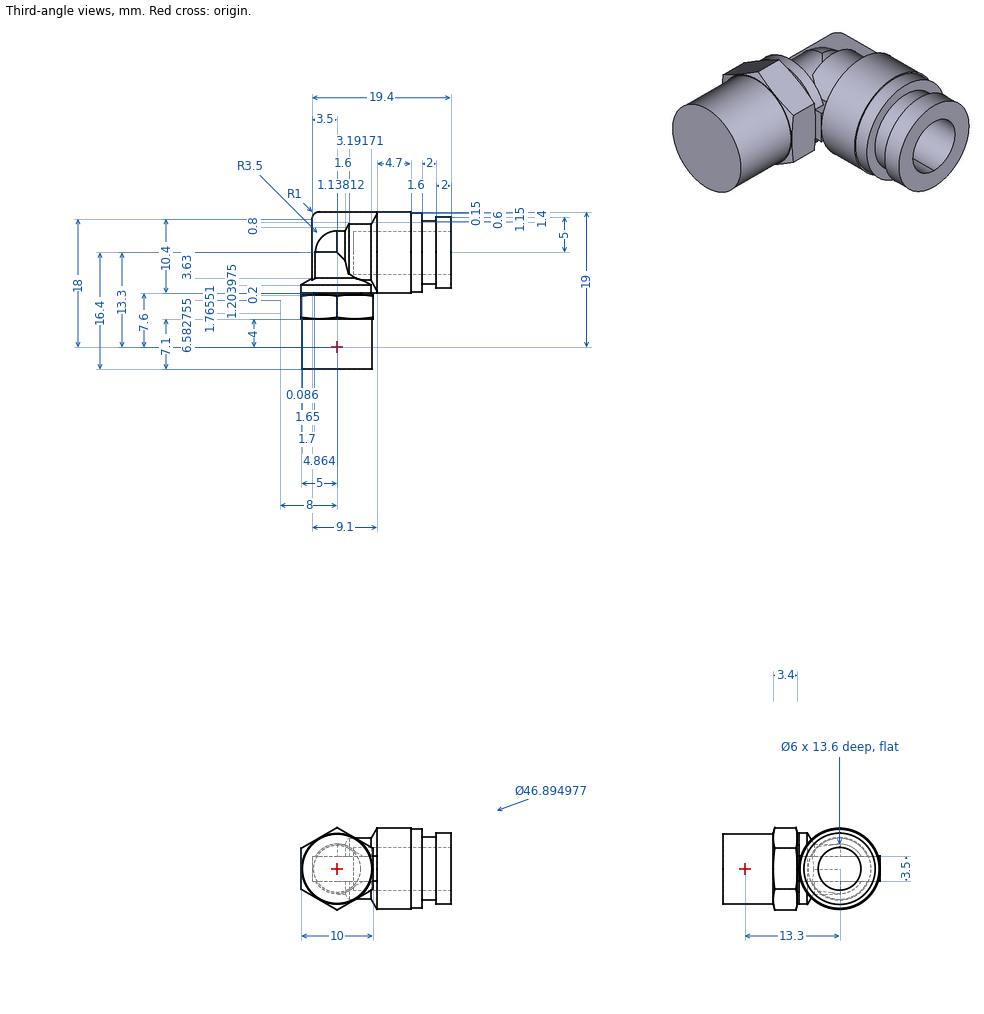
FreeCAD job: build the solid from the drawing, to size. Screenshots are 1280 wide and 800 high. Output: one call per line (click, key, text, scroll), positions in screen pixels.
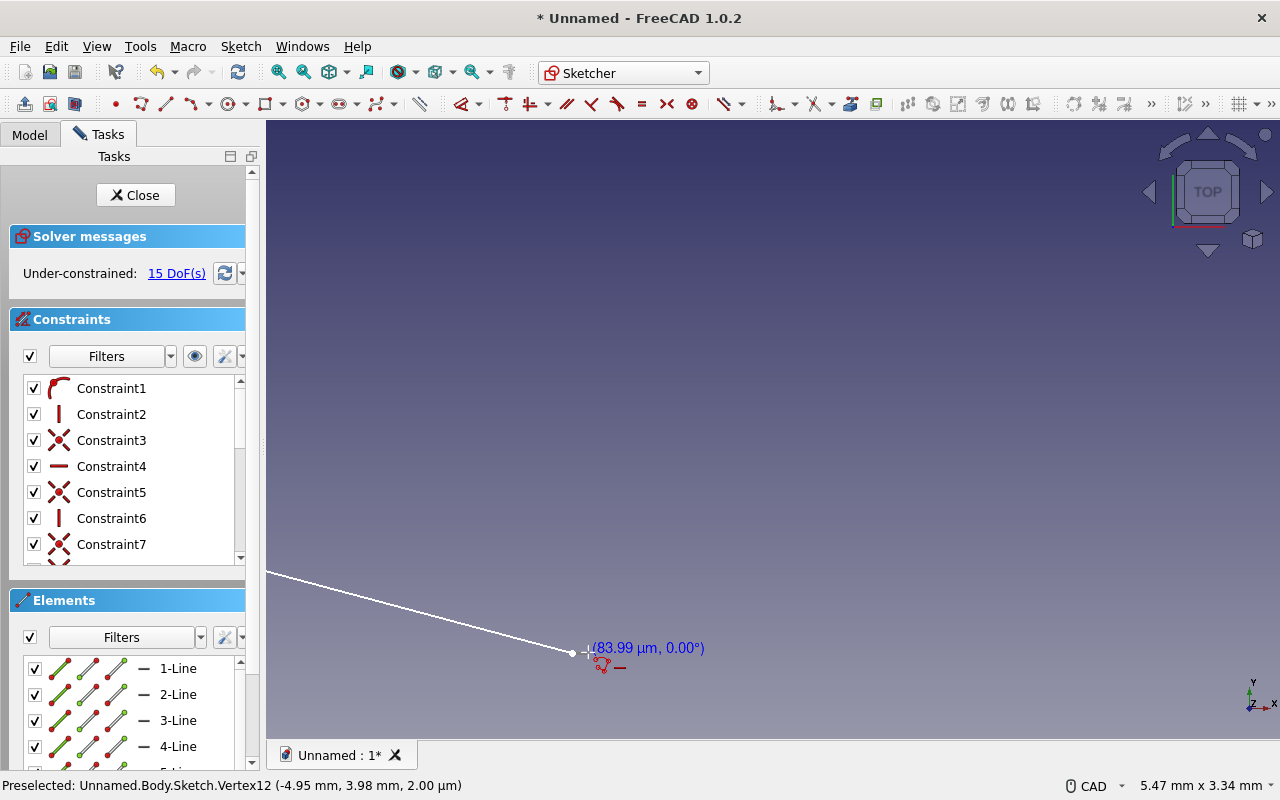
click(588, 651)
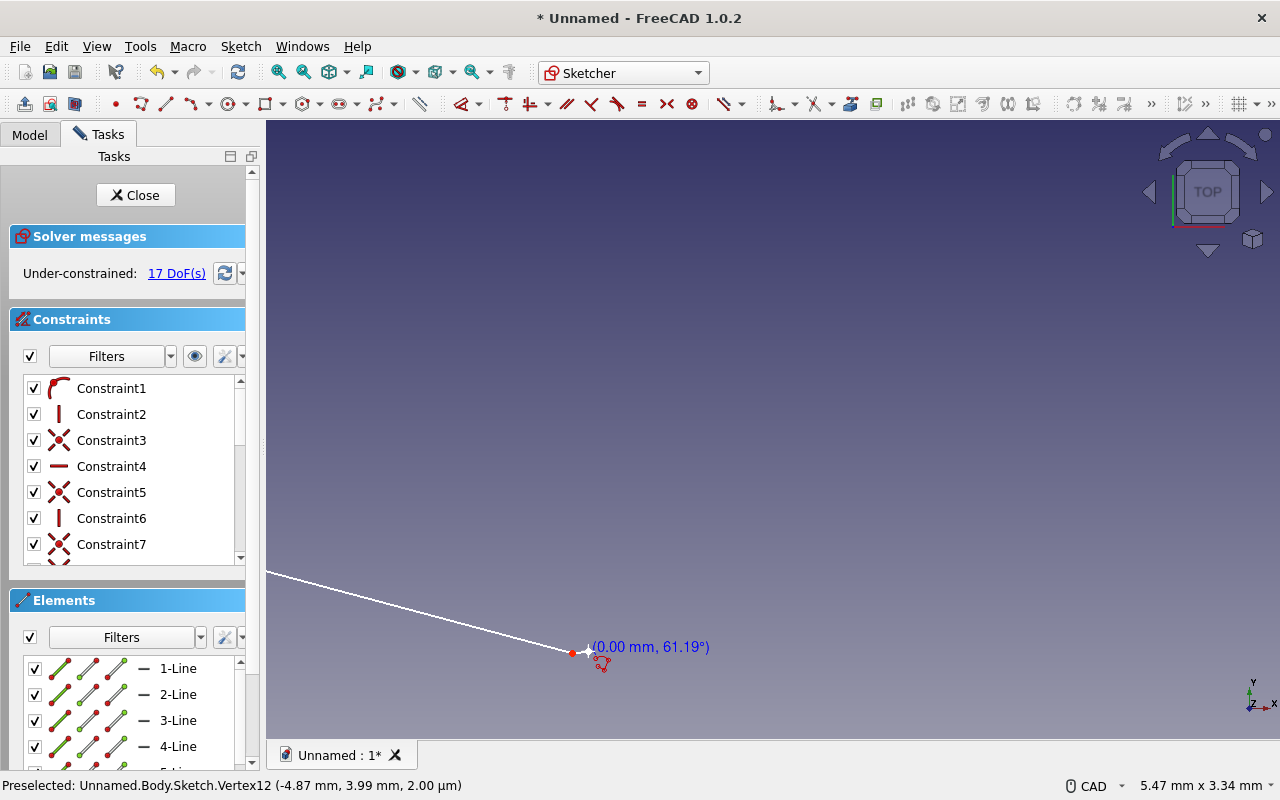
scroll(698, 427, down, 10)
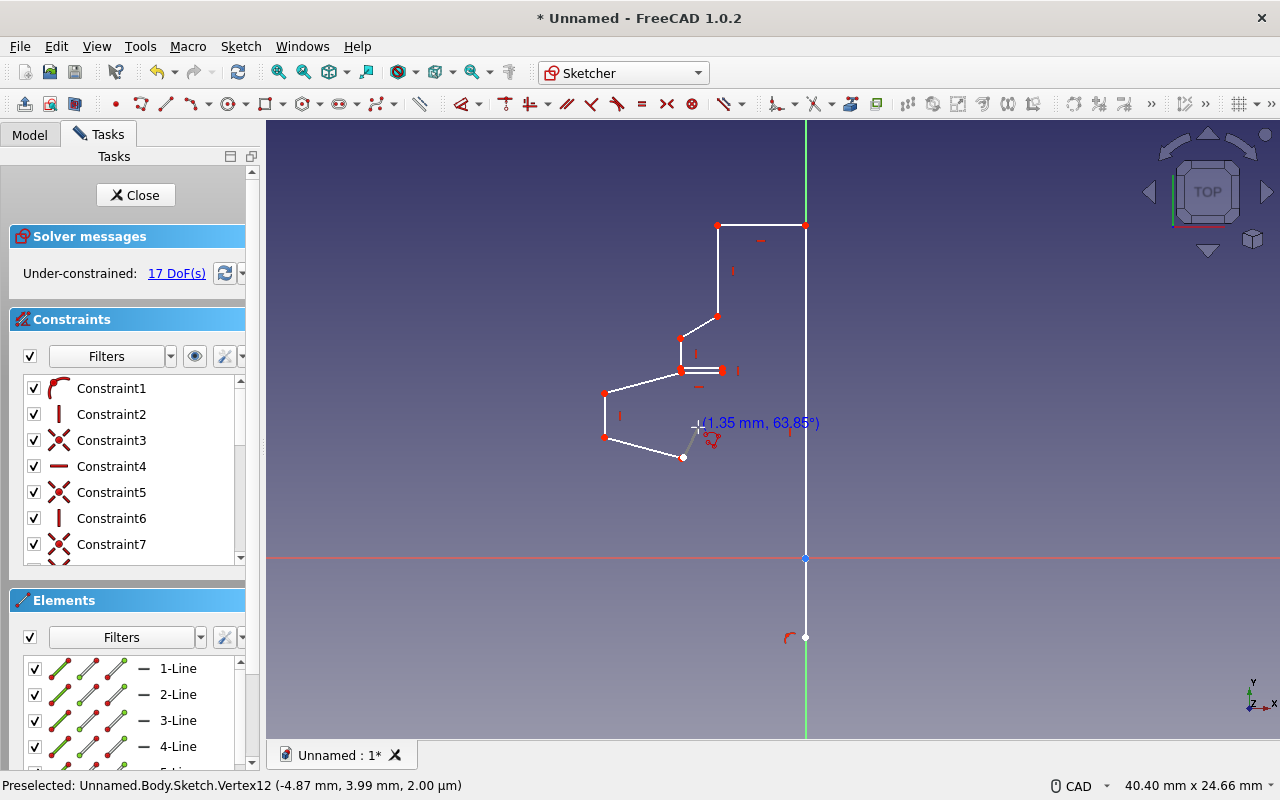
click(683, 636)
click(806, 637)
key(Escape)
key(Escape)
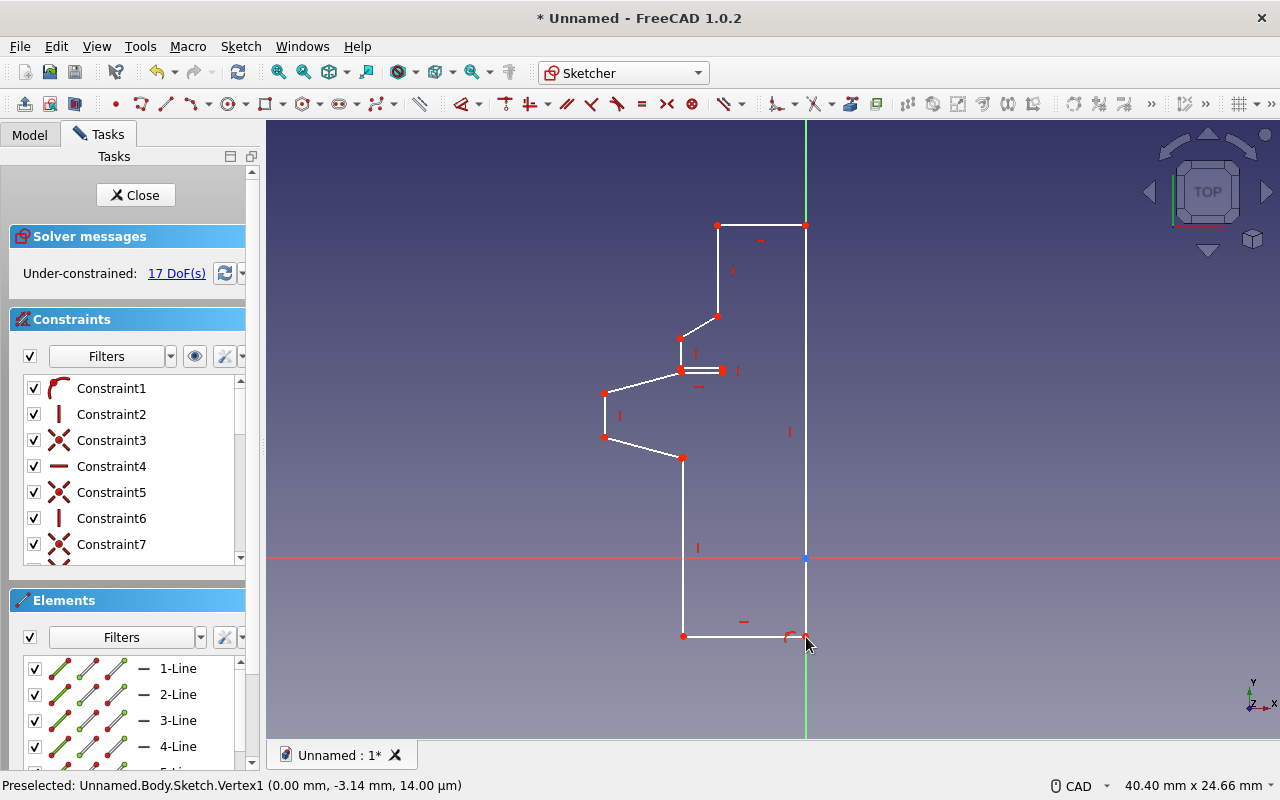
scroll(682, 458, up, 13)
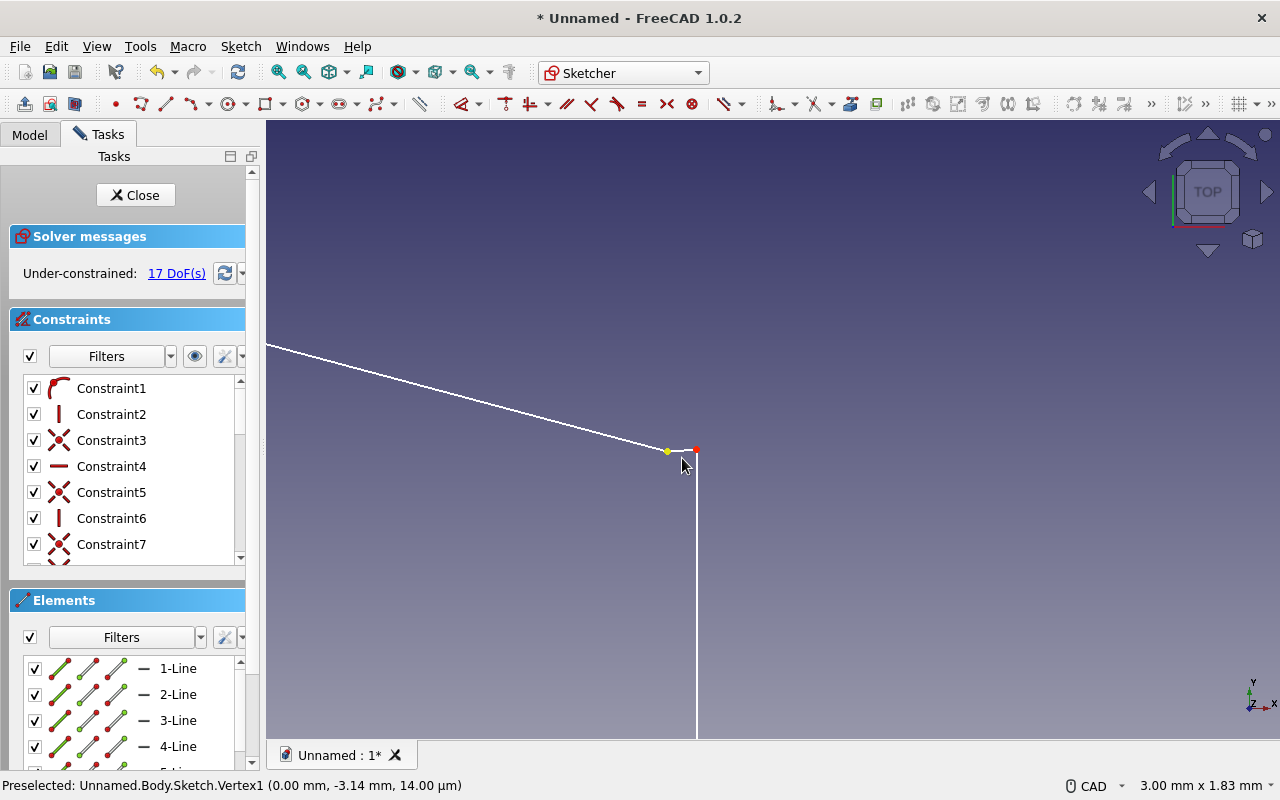
click(682, 451)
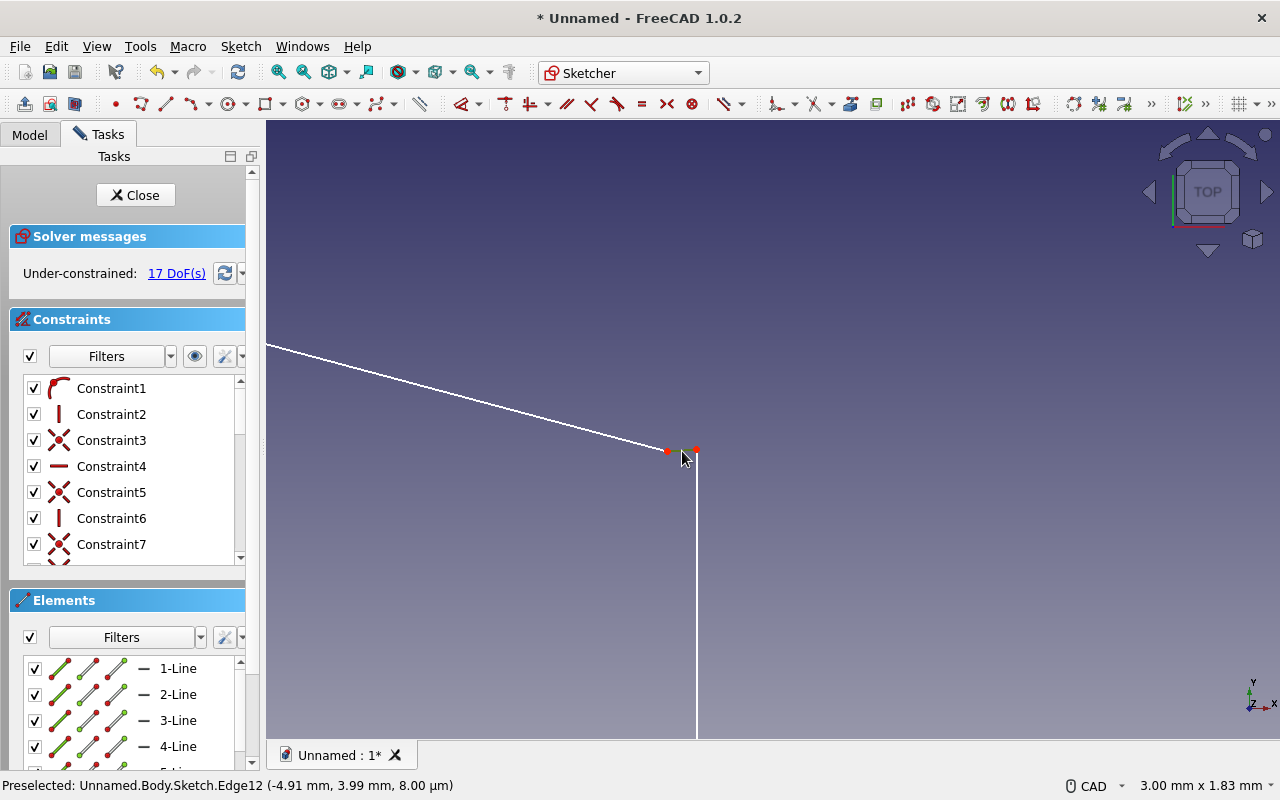
key(h)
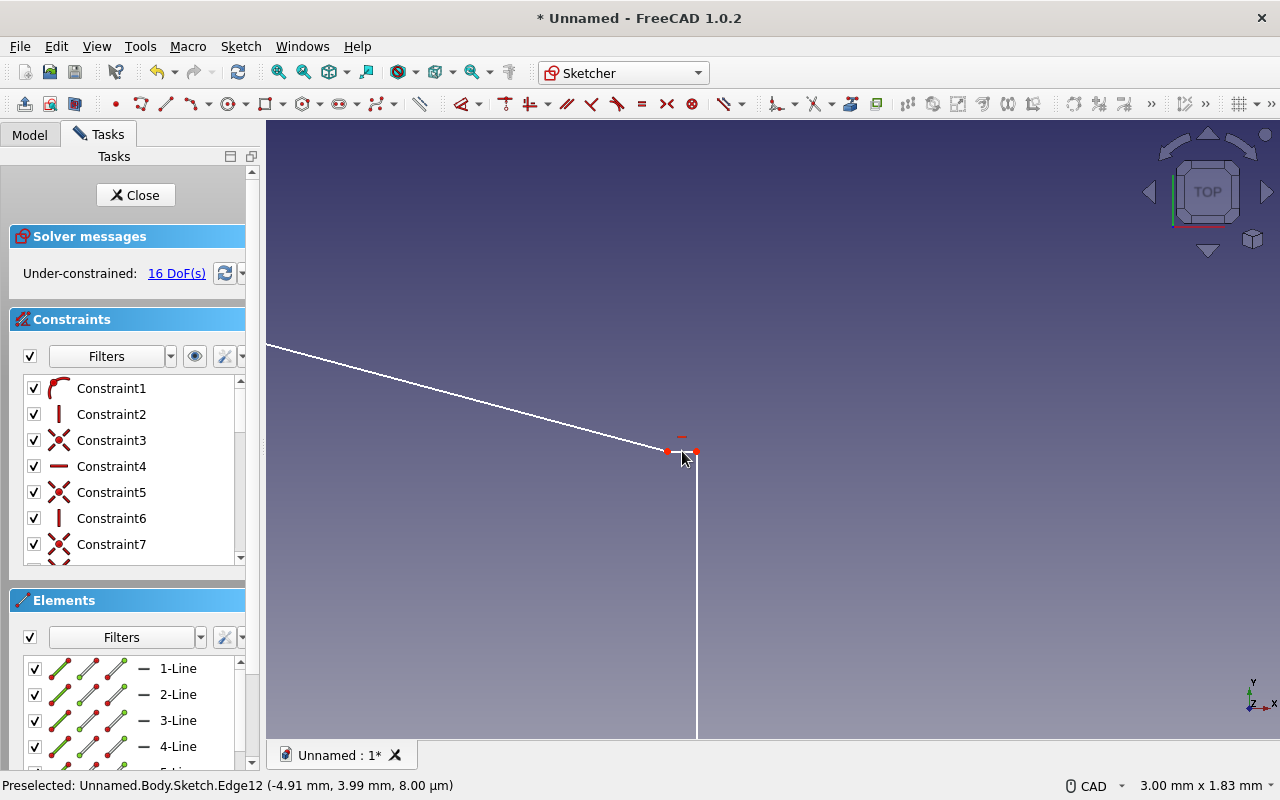
scroll(682, 458, down, 13)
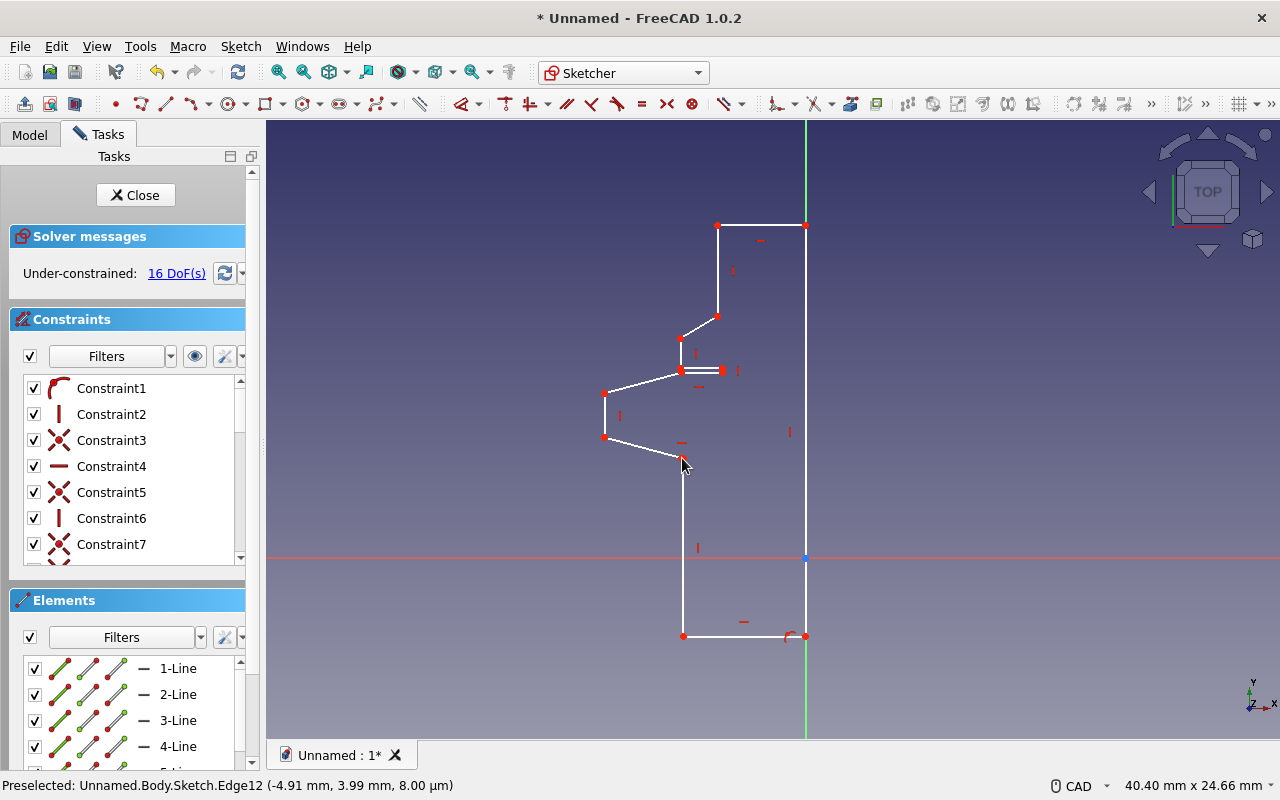
click(681, 338)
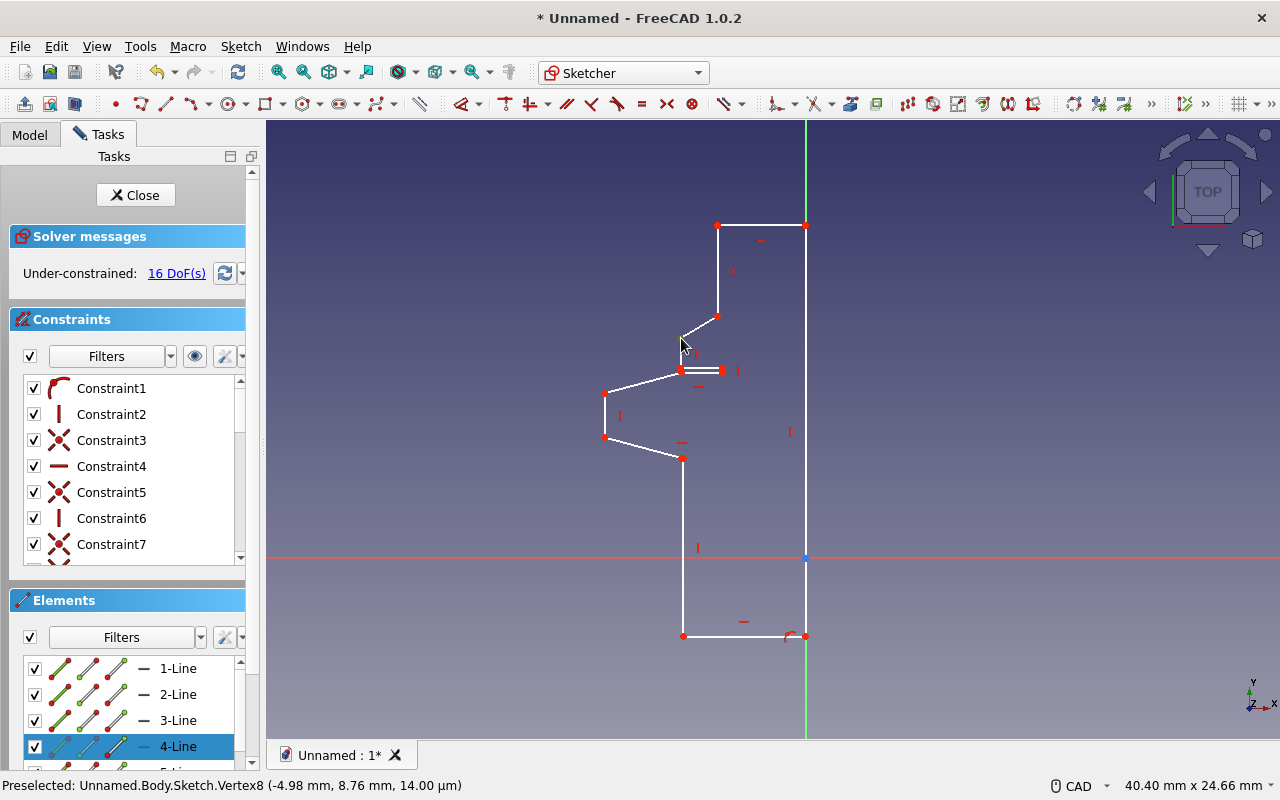
key(l)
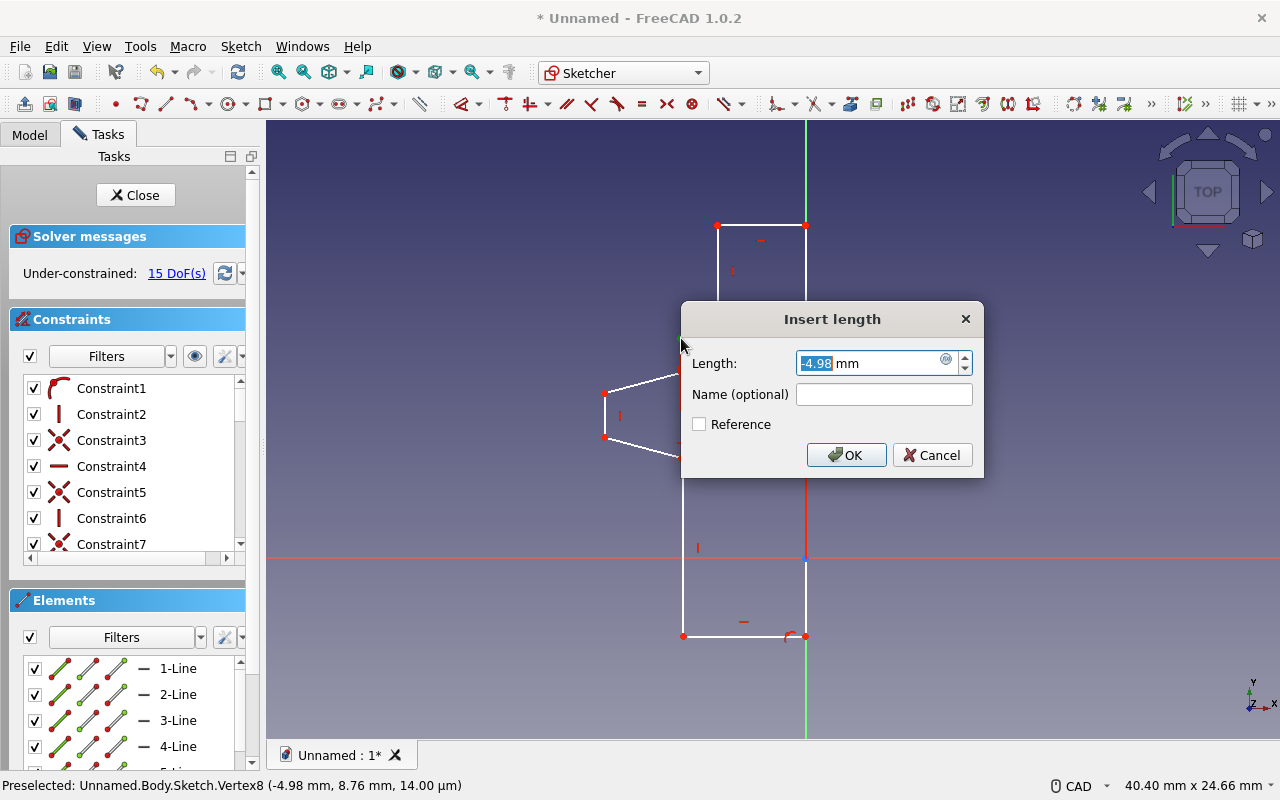
text(-5)
key(Return)